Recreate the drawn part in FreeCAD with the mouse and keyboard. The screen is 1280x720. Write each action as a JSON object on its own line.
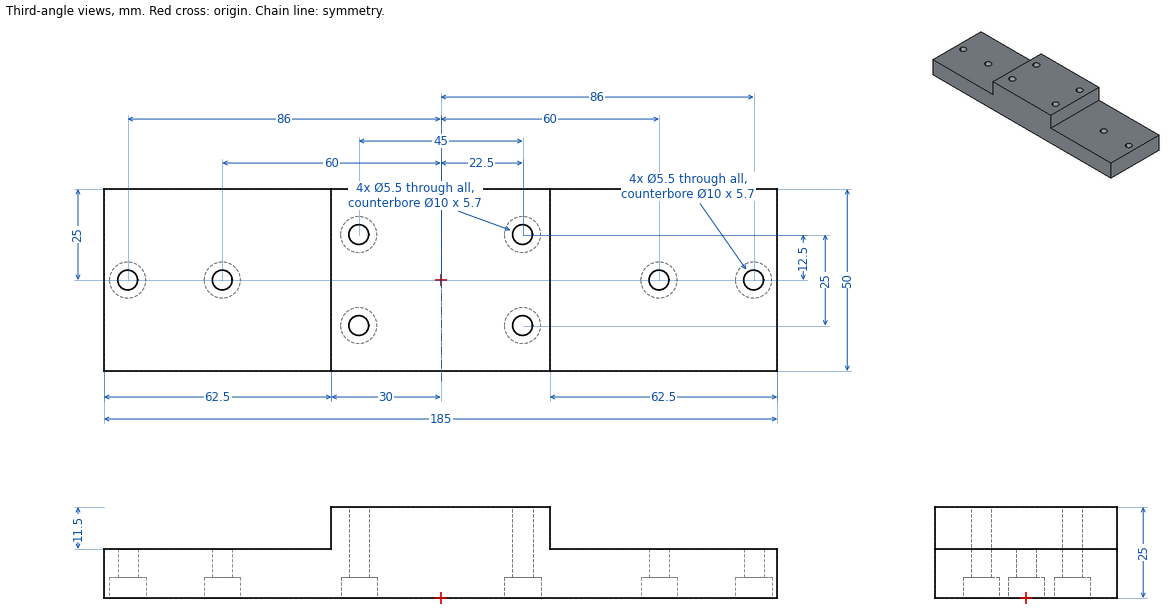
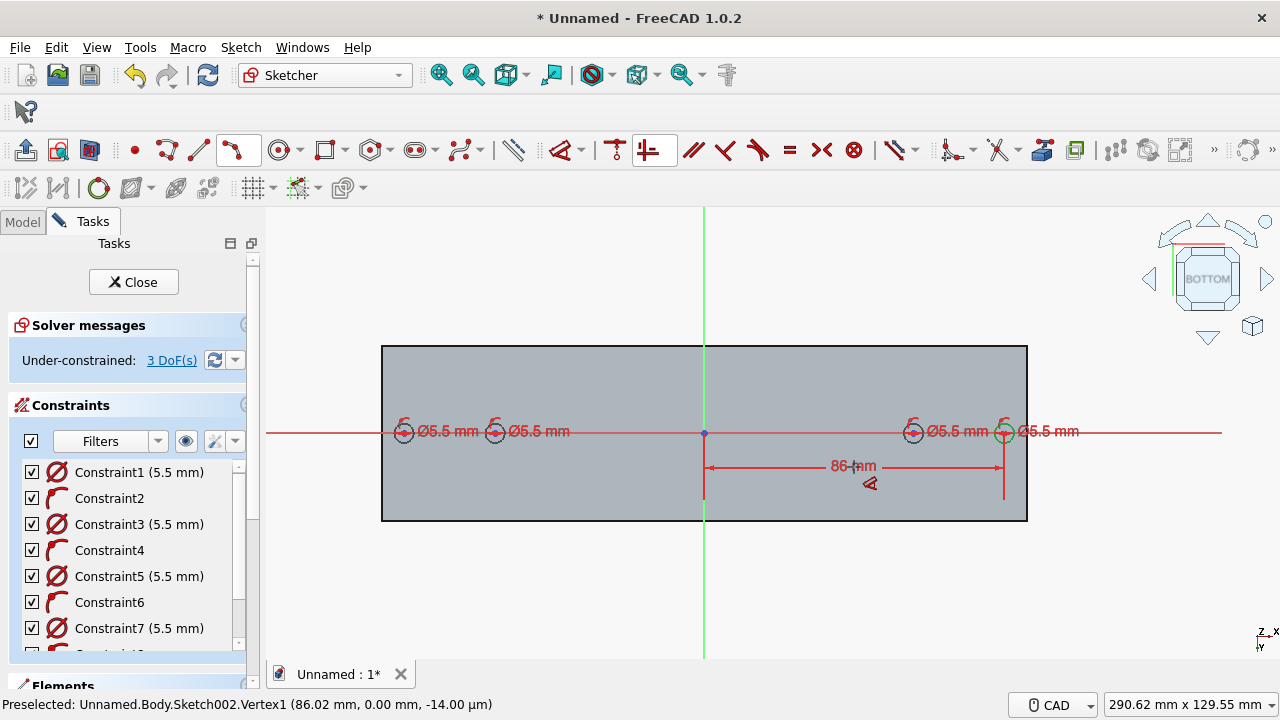
{"action": "left_click", "coordinate": [914, 433]}
{"action": "left_click", "coordinate": [761, 467]}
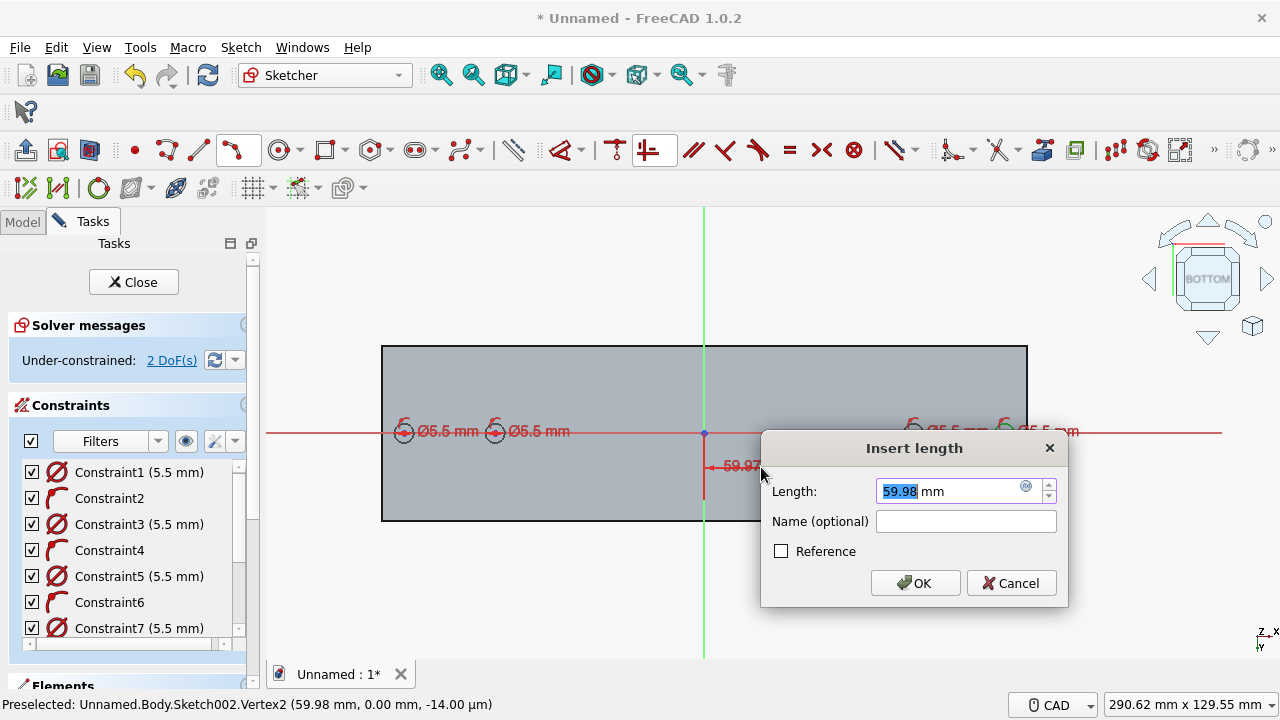
{"action": "type", "text": "60"}
{"action": "key", "text": "Return"}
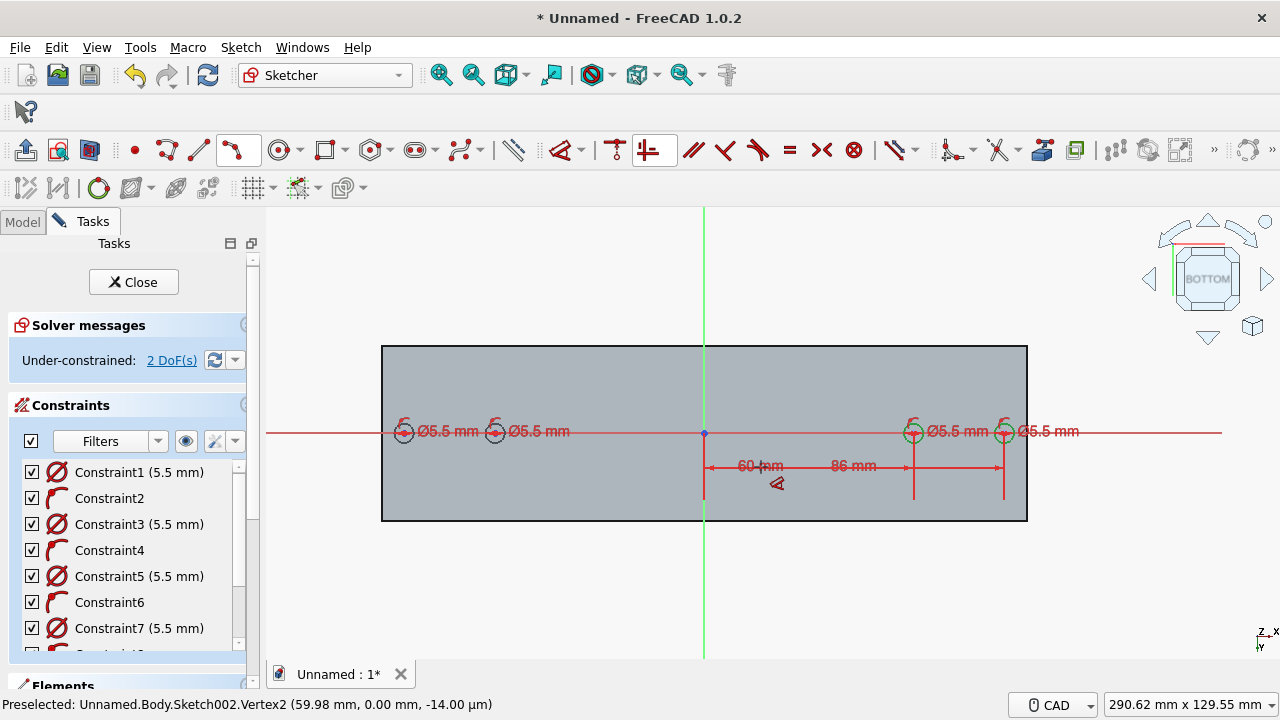
{"action": "left_click", "coordinate": [495, 433]}
{"action": "left_click", "coordinate": [600, 467]}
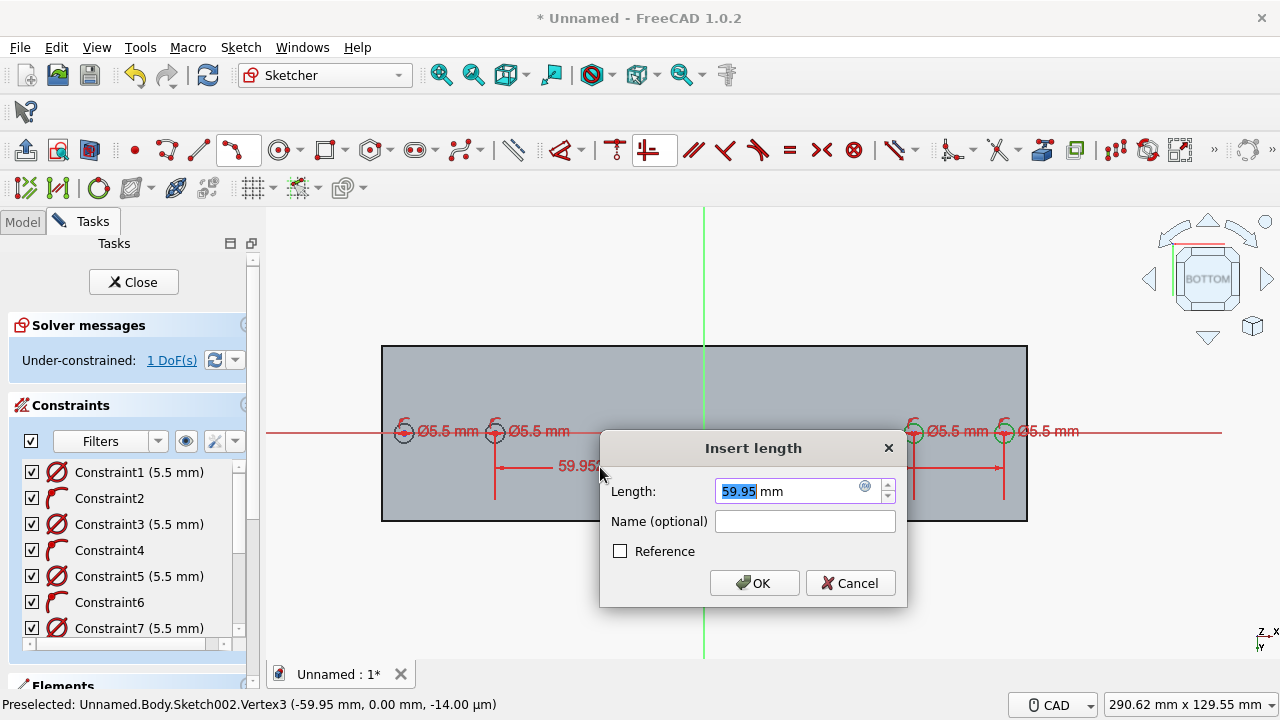
{"action": "type", "text": "60"}
{"action": "key", "text": "Return"}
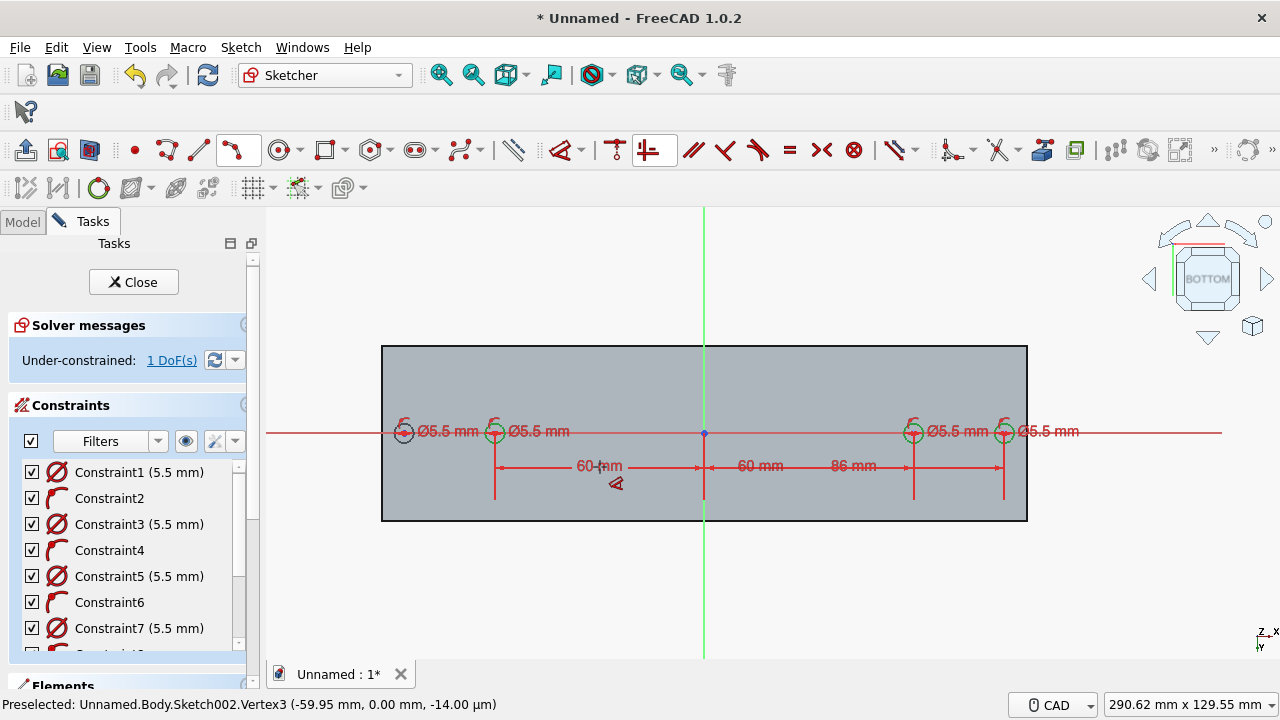
{"action": "left_click", "coordinate": [404, 433]}
{"action": "left_click", "coordinate": [485, 467]}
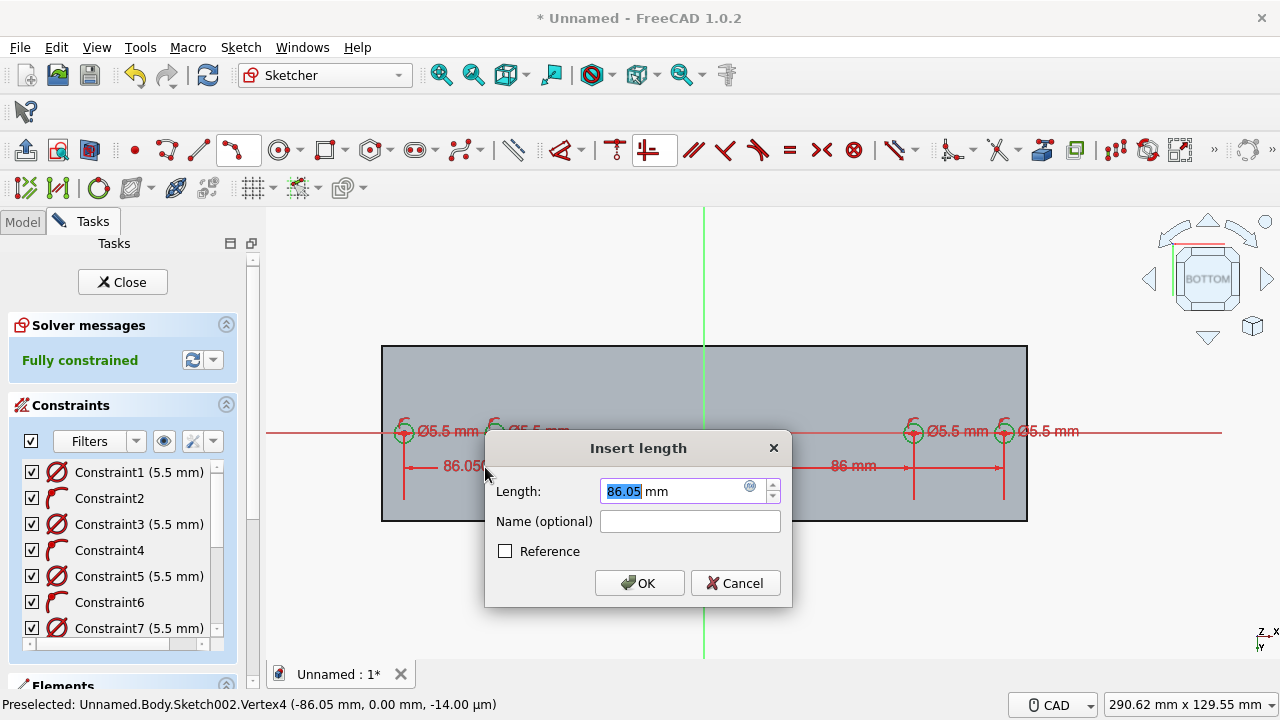
{"action": "type", "text": "86"}
{"action": "key", "text": "Return"}
{"action": "key", "text": "Escape"}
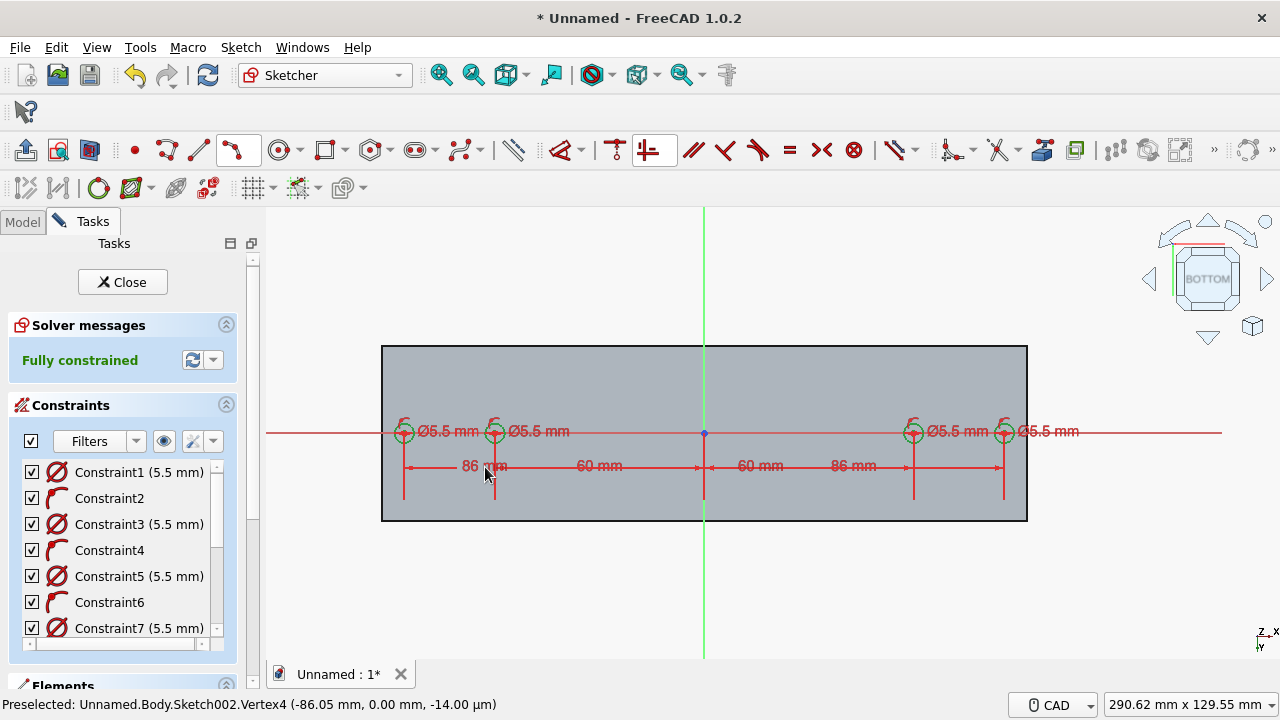
{"action": "left_click", "coordinate": [123, 282]}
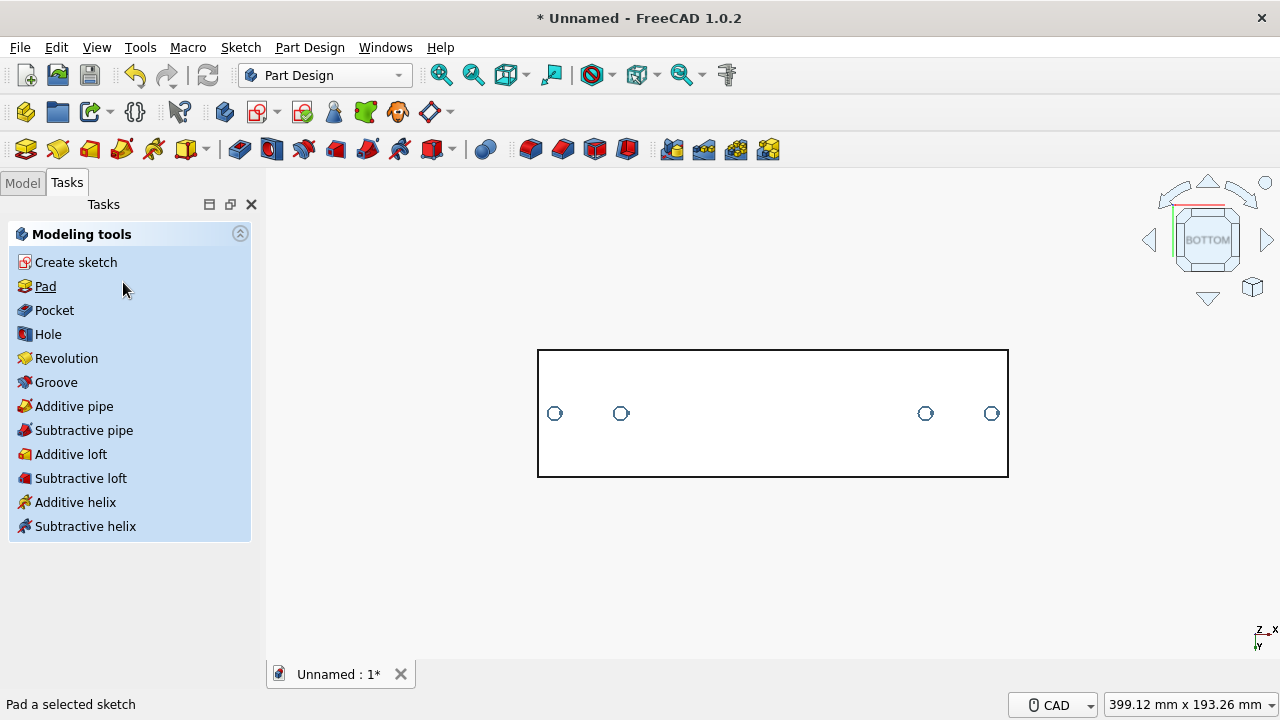
{"action": "left_click", "coordinate": [272, 150]}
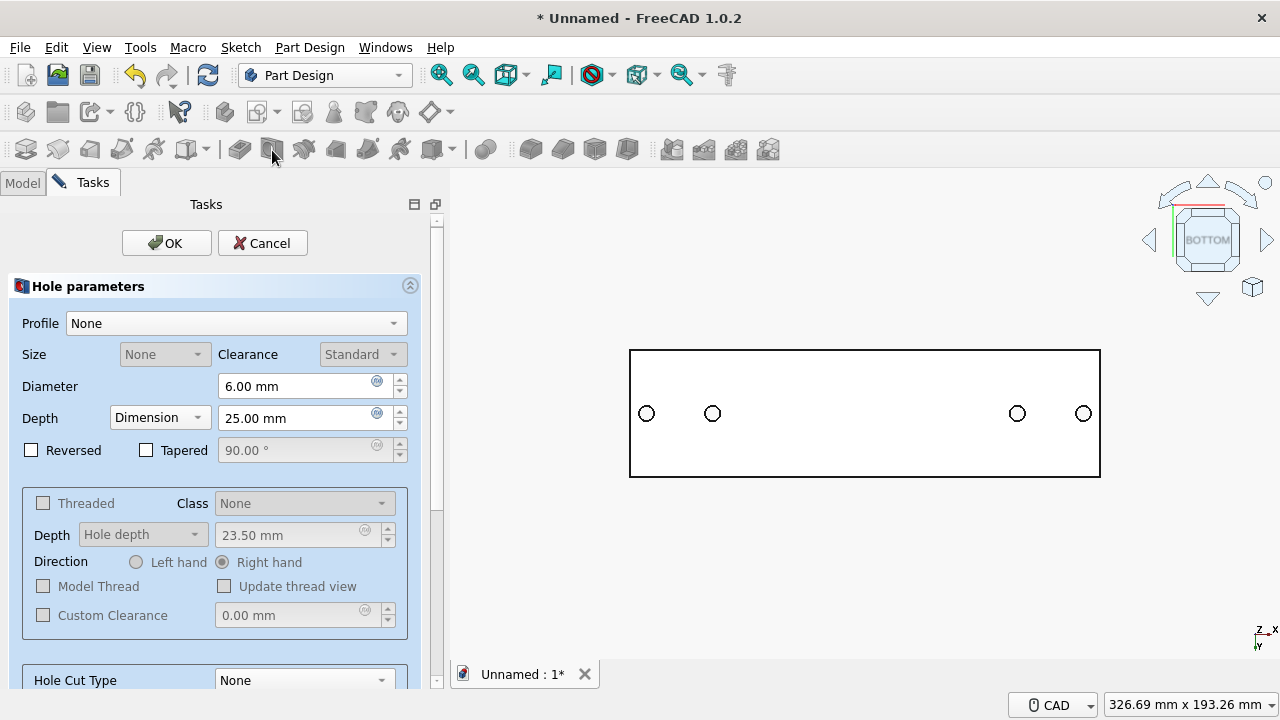
{"action": "triple_click", "coordinate": [305, 386]}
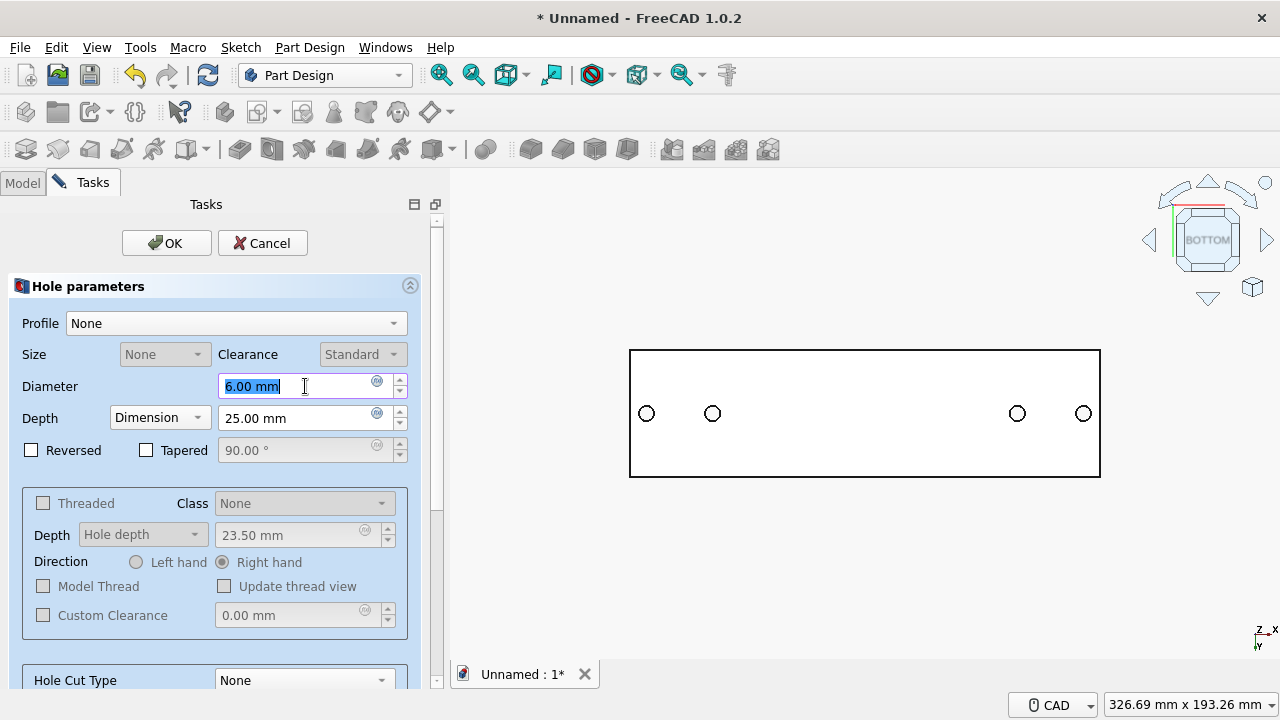
{"action": "type", "text": "5.5"}
{"action": "key", "text": "Tab"}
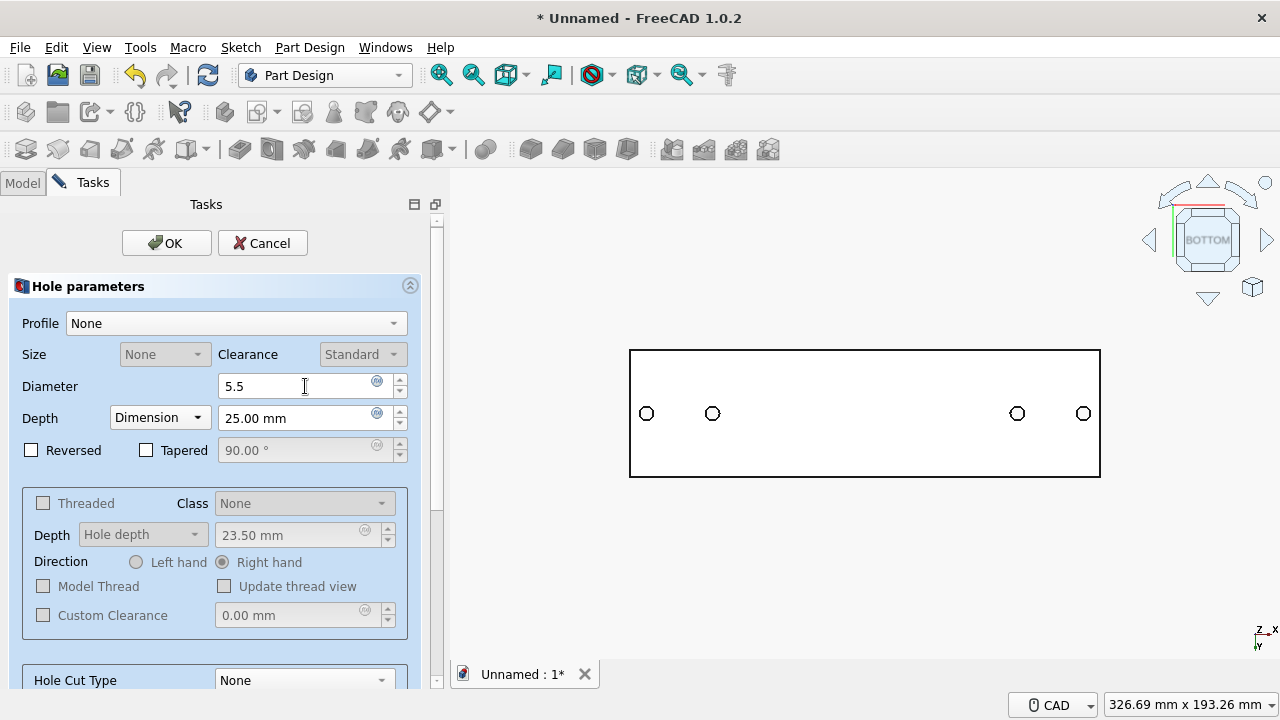
{"action": "left_click", "coordinate": [161, 418]}